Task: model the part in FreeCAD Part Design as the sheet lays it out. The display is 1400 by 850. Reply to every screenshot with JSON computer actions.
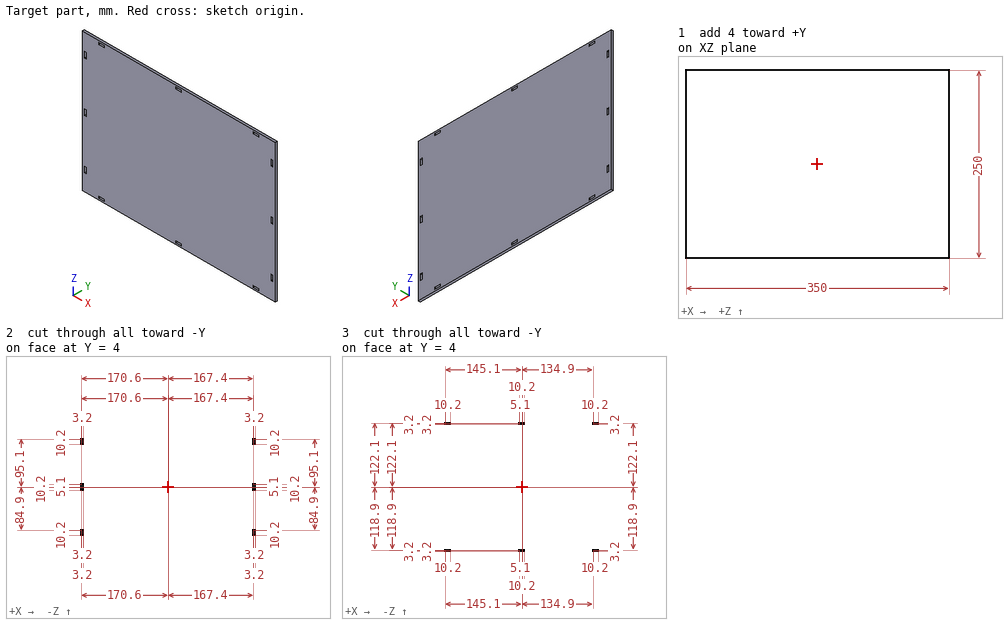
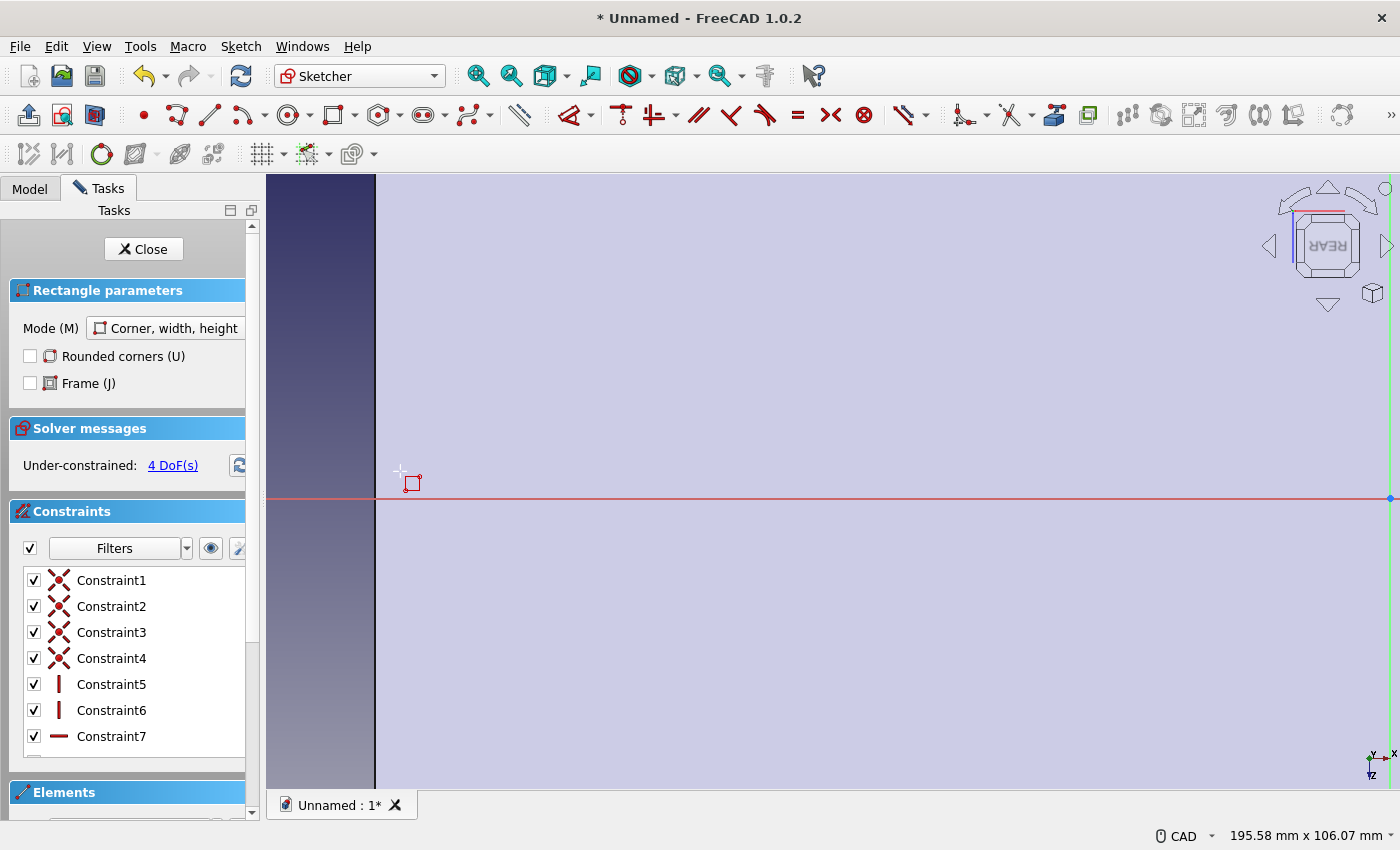
{"action": "left_click", "coordinate": [401, 469]}
{"action": "left_click", "coordinate": [420, 528]}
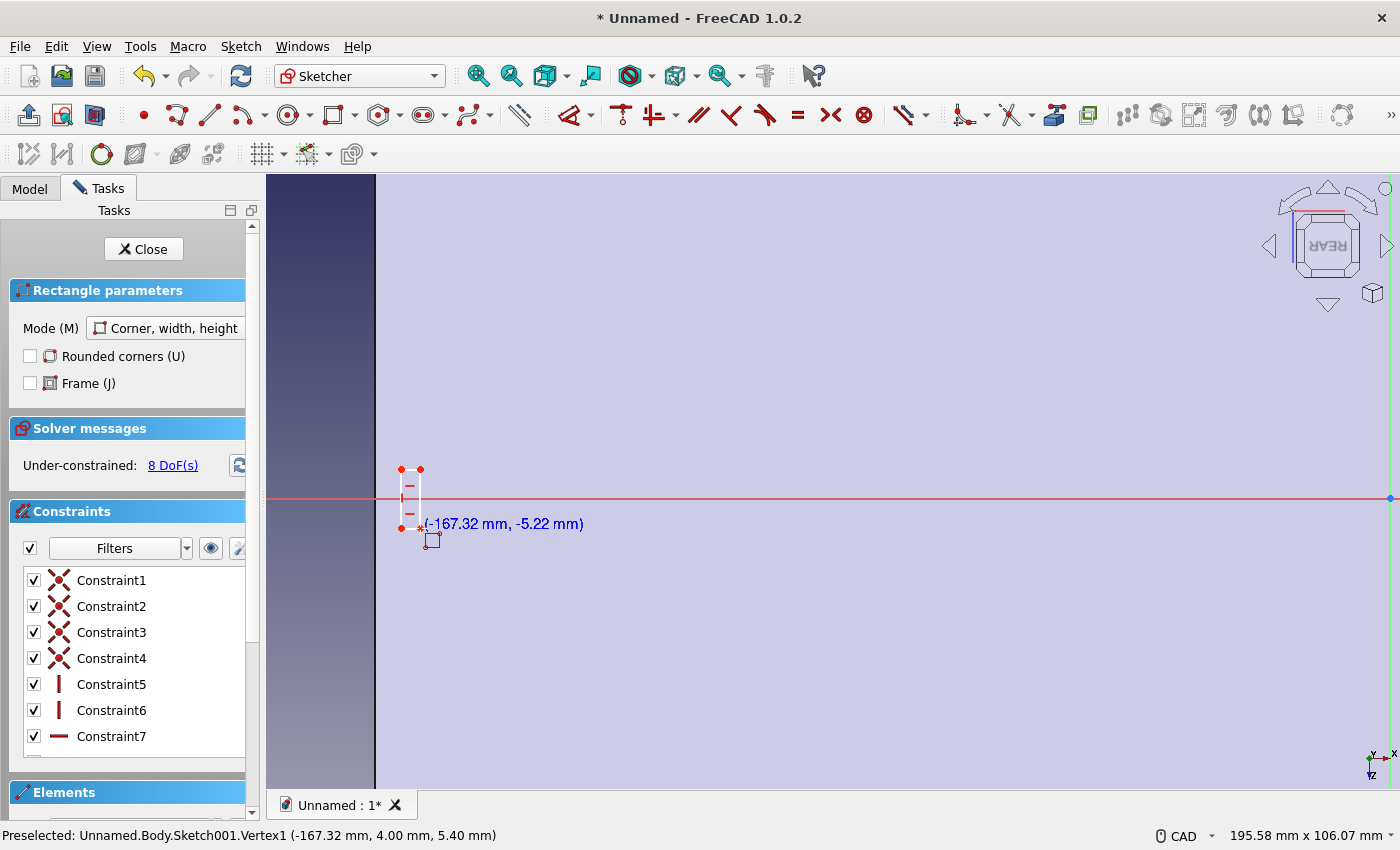
{"action": "scroll", "coordinate": [400, 471], "scroll_direction": "down", "scroll_amount": 5}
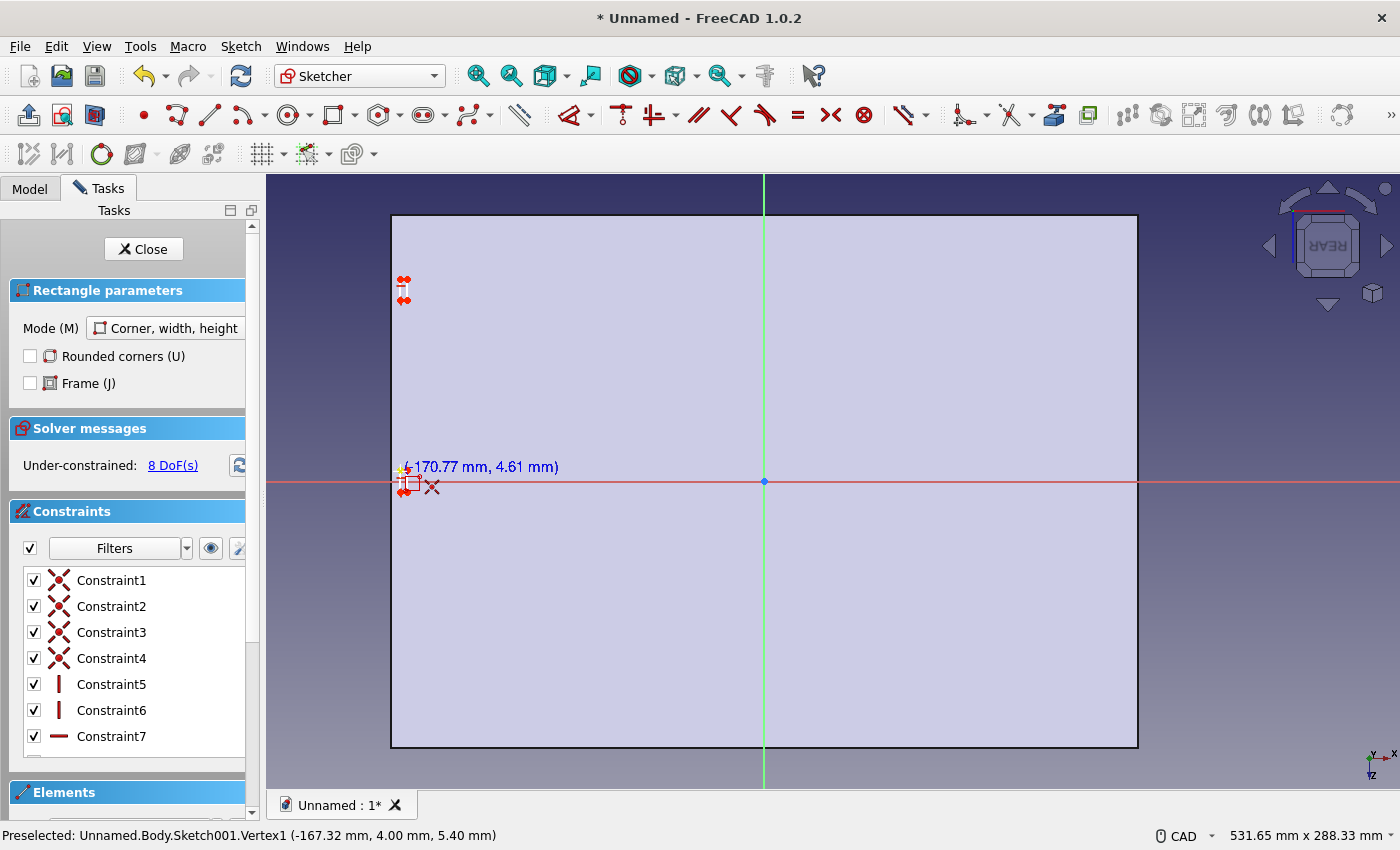
{"action": "scroll", "coordinate": [400, 663], "scroll_direction": "up", "scroll_amount": 5}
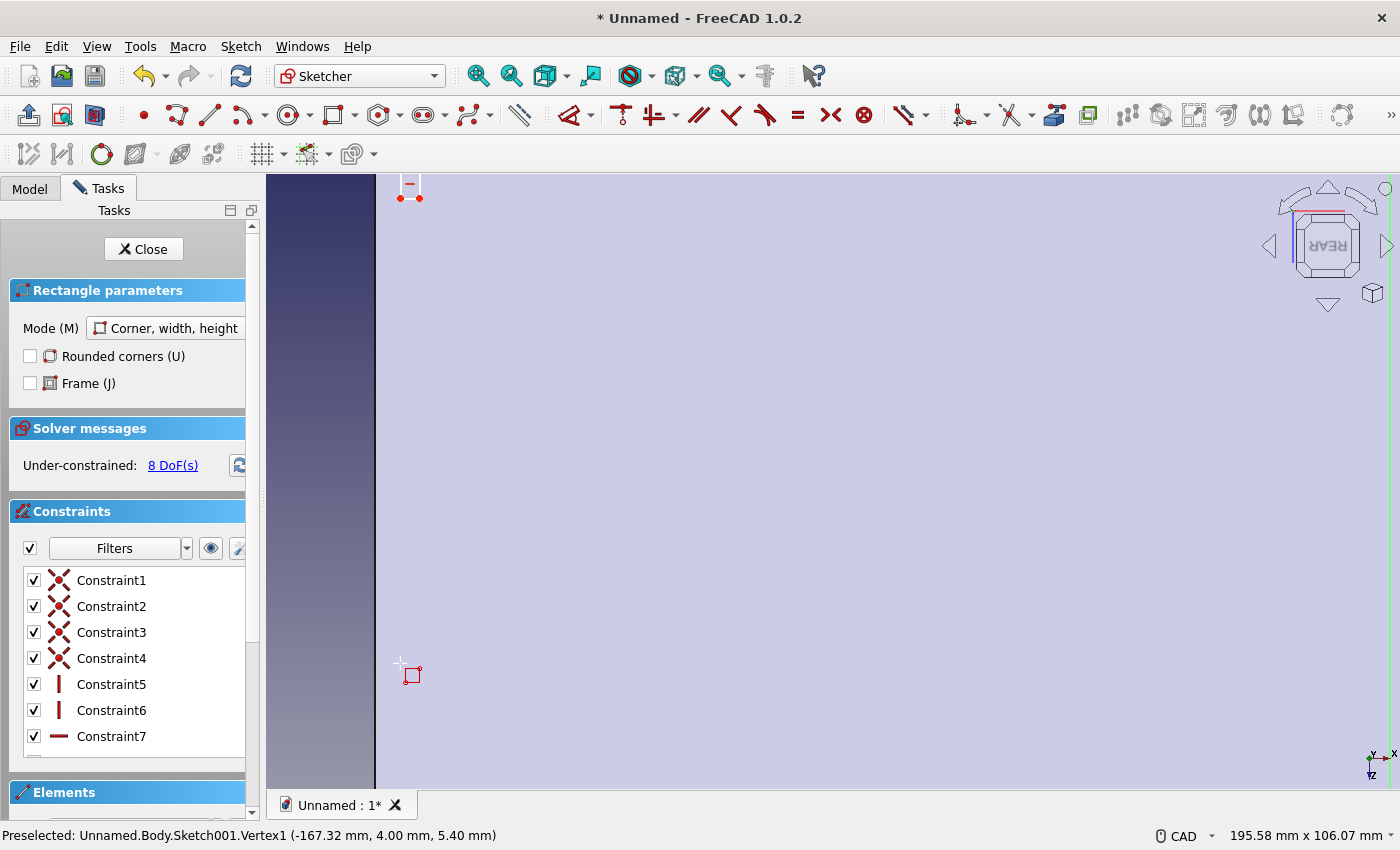
{"action": "left_click", "coordinate": [401, 661]}
{"action": "left_click", "coordinate": [420, 720]}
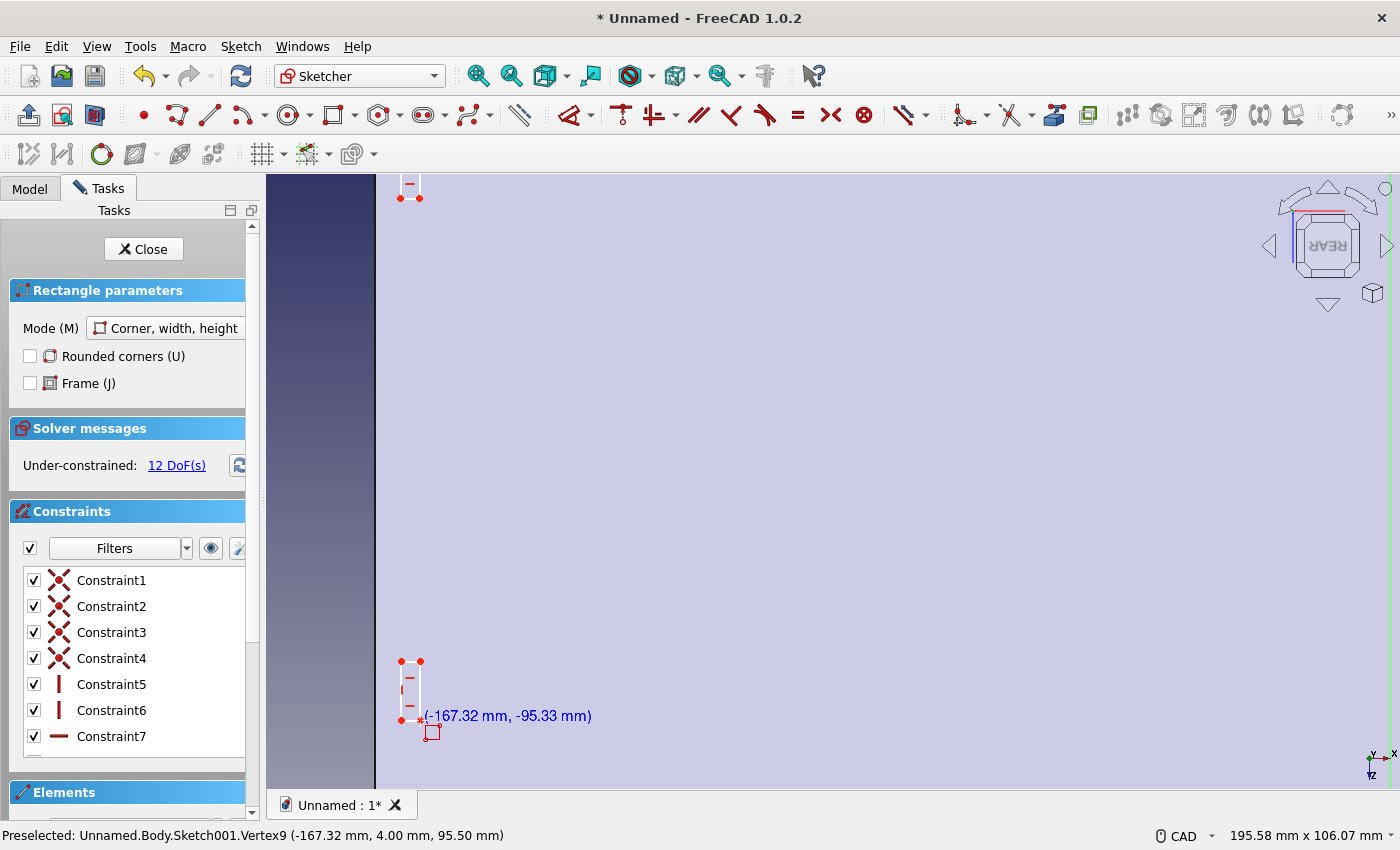
{"action": "scroll", "coordinate": [400, 664], "scroll_direction": "down", "scroll_amount": 5}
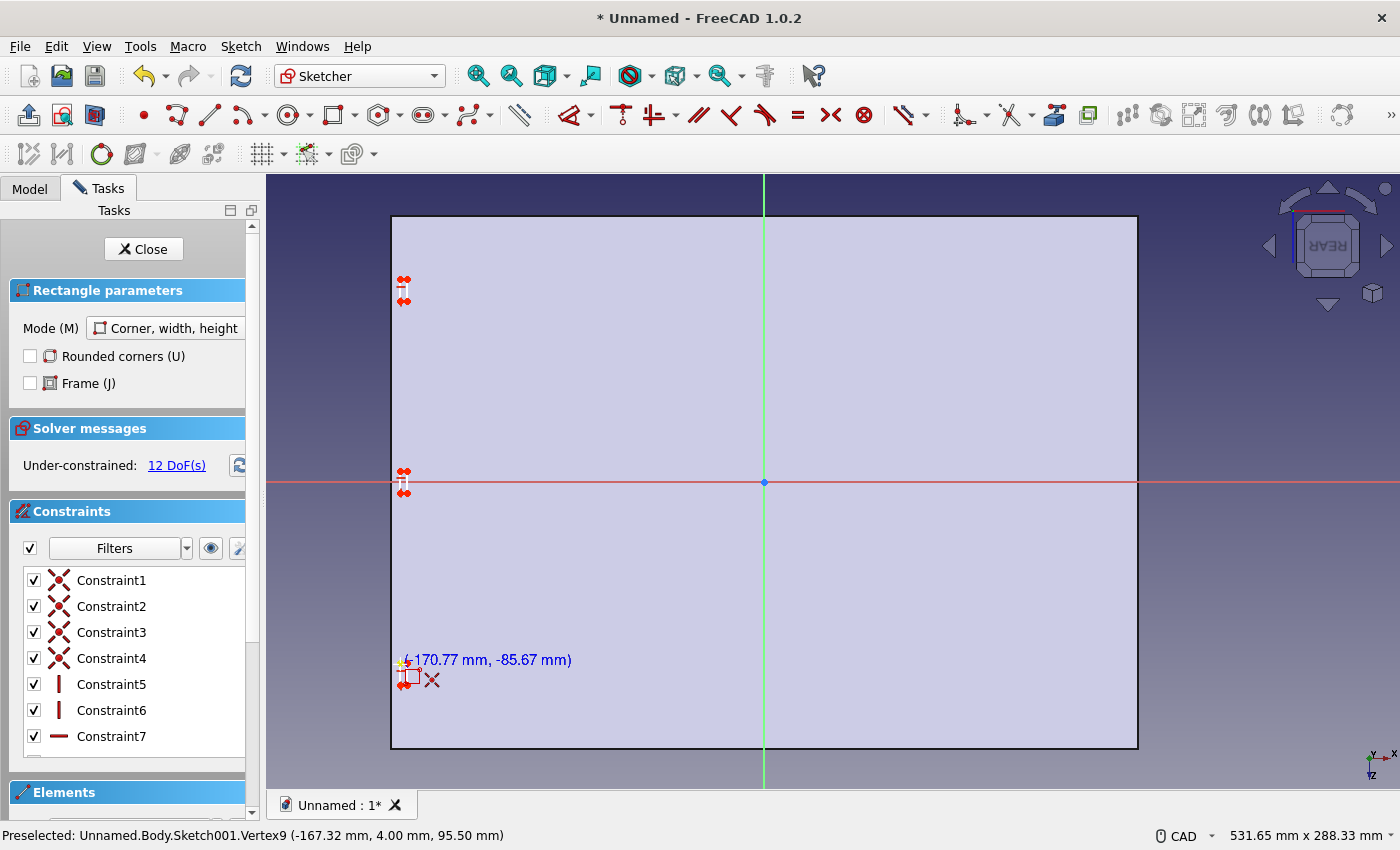
{"action": "scroll", "coordinate": [1121, 663], "scroll_direction": "up", "scroll_amount": 5}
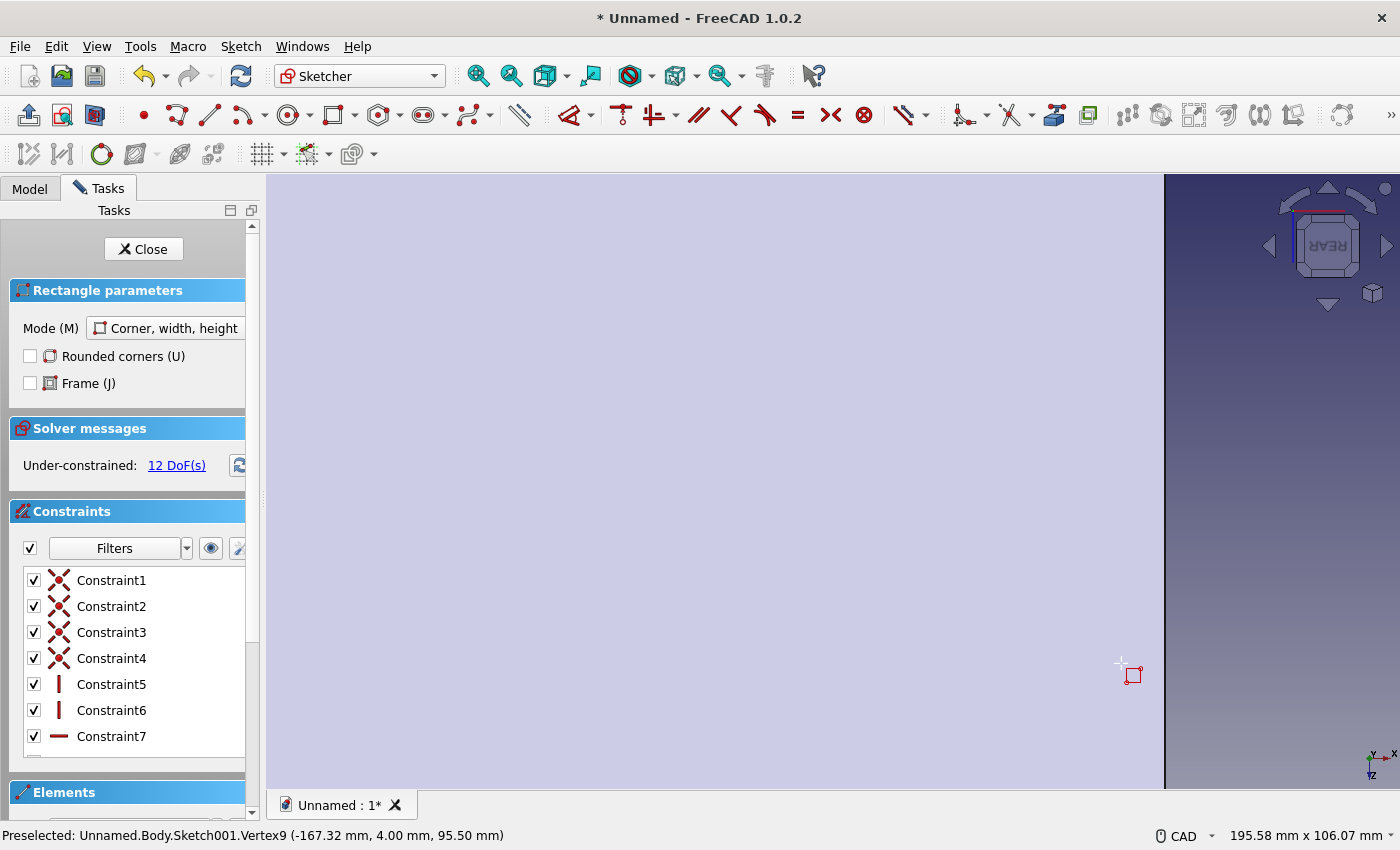
{"action": "left_click", "coordinate": [1121, 662]}
{"action": "left_click", "coordinate": [1139, 721]}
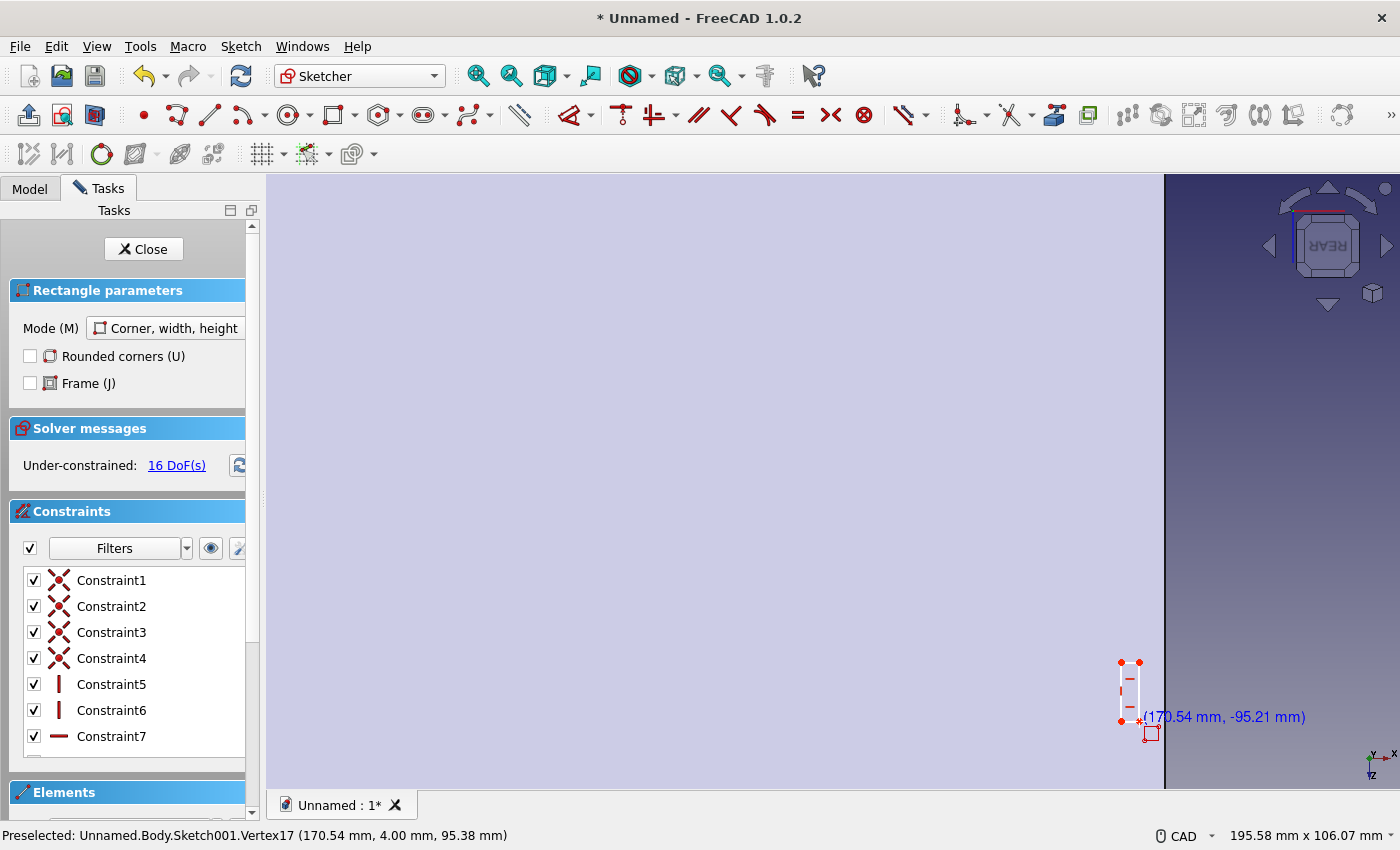
{"action": "scroll", "coordinate": [1122, 663], "scroll_direction": "down", "scroll_amount": 5}